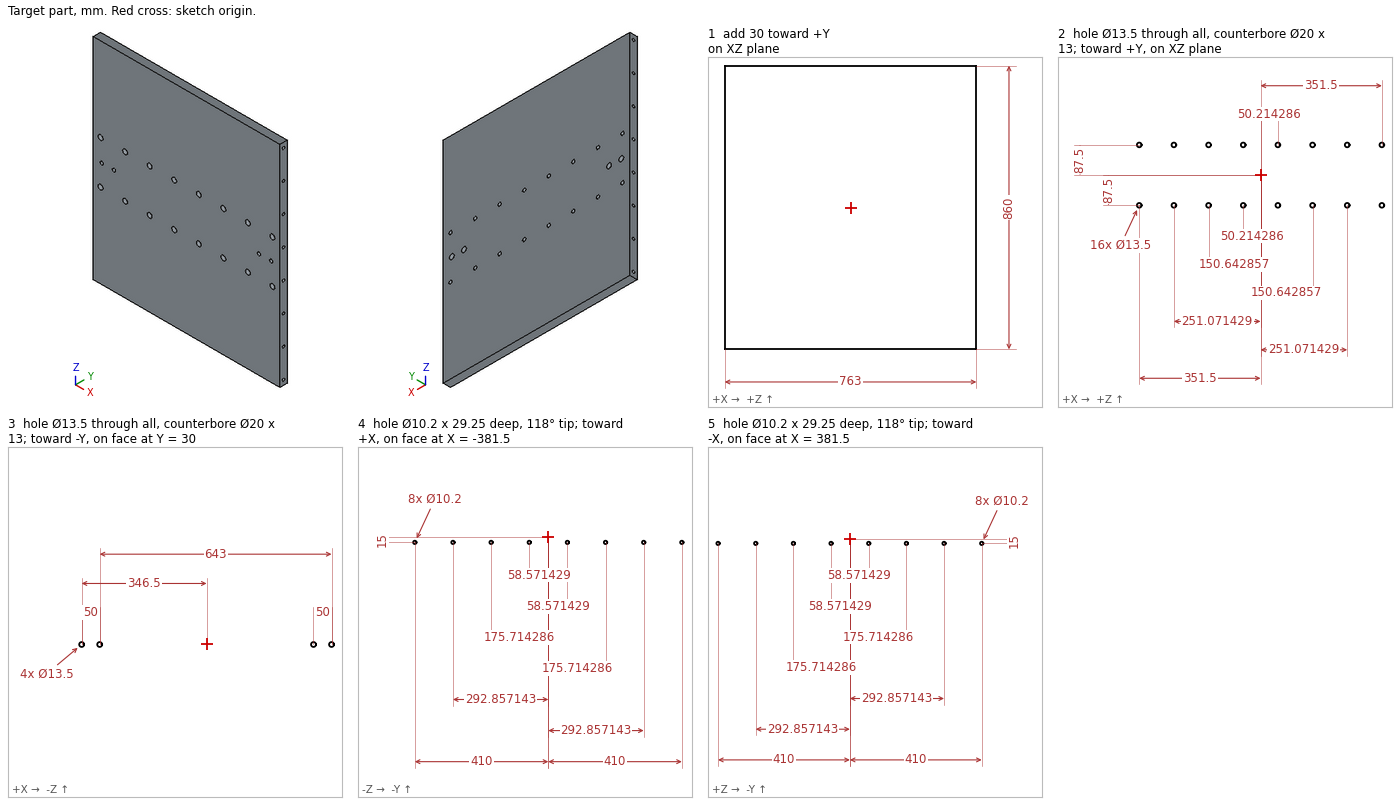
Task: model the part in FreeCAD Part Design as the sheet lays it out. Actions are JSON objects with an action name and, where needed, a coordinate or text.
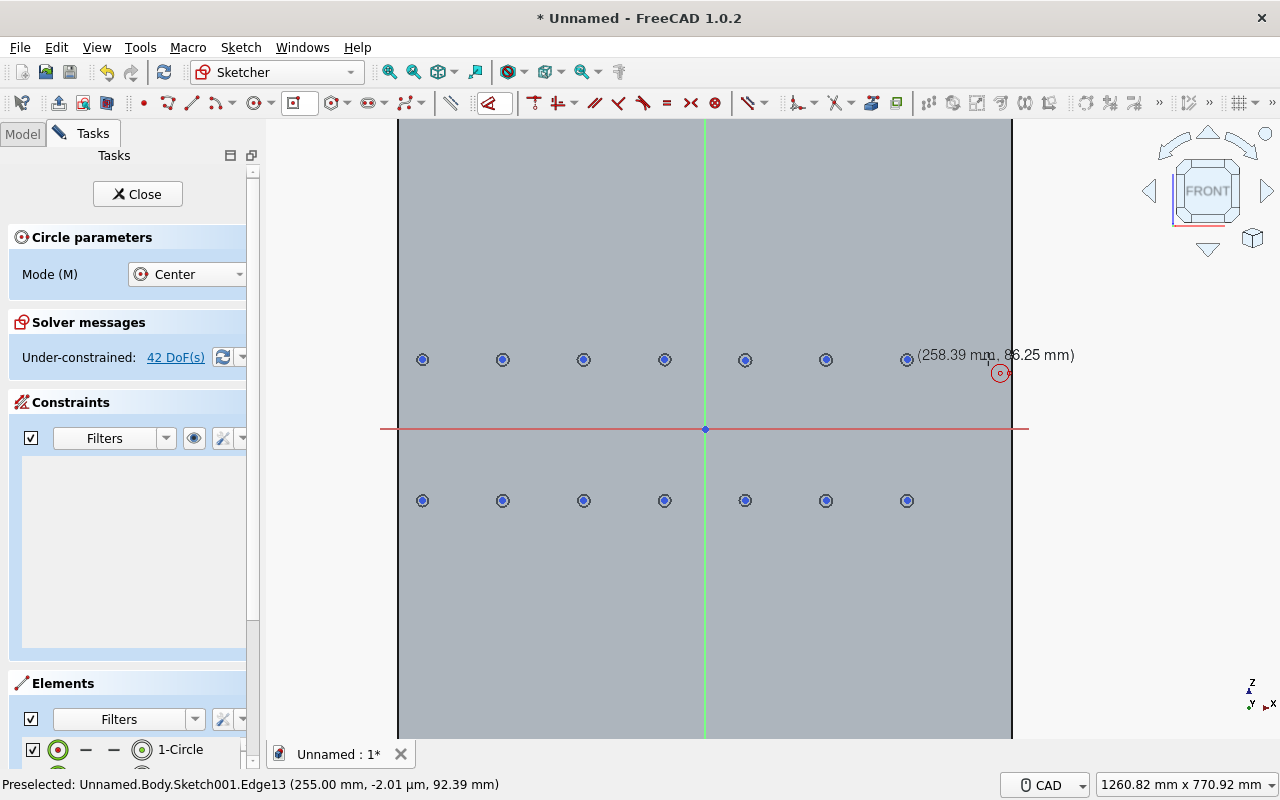
{"action": "left_click", "coordinate": [988, 359]}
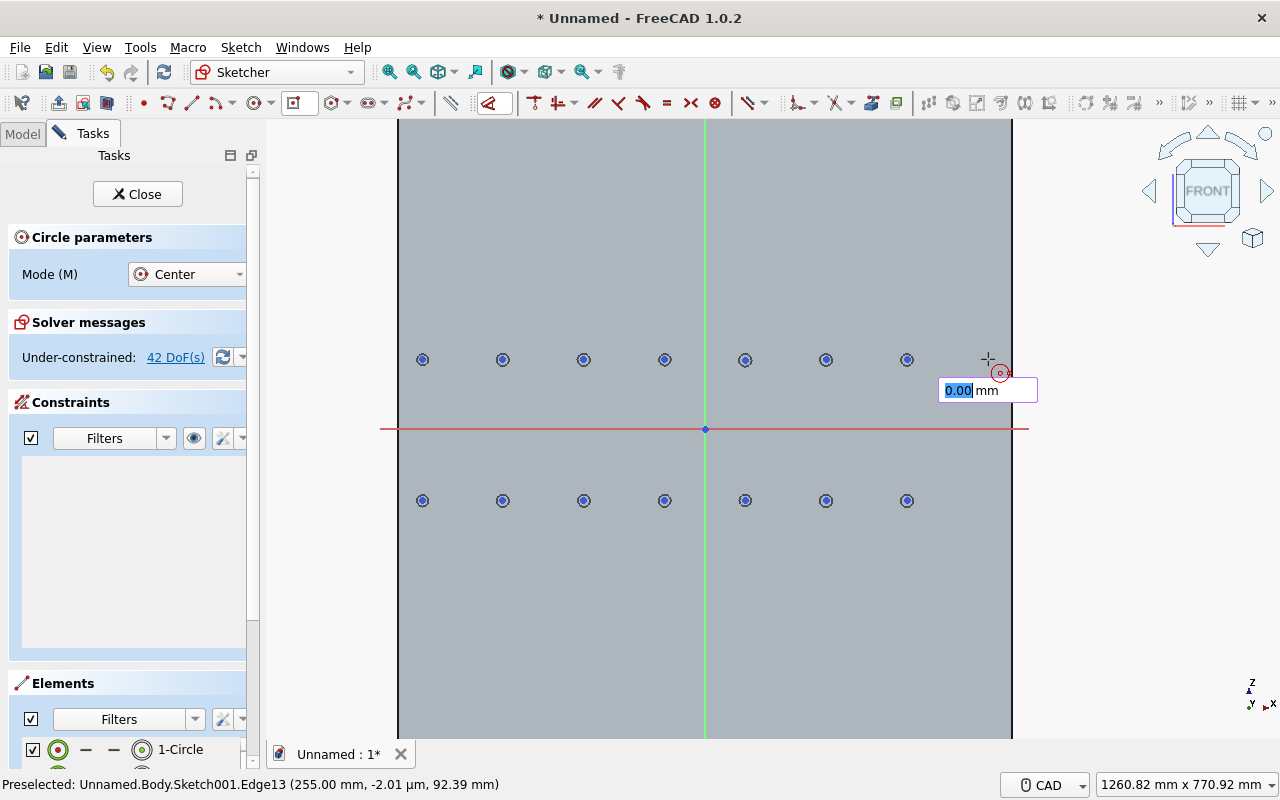
{"action": "scroll", "coordinate": [992, 355], "scroll_direction": "up", "scroll_amount": 6}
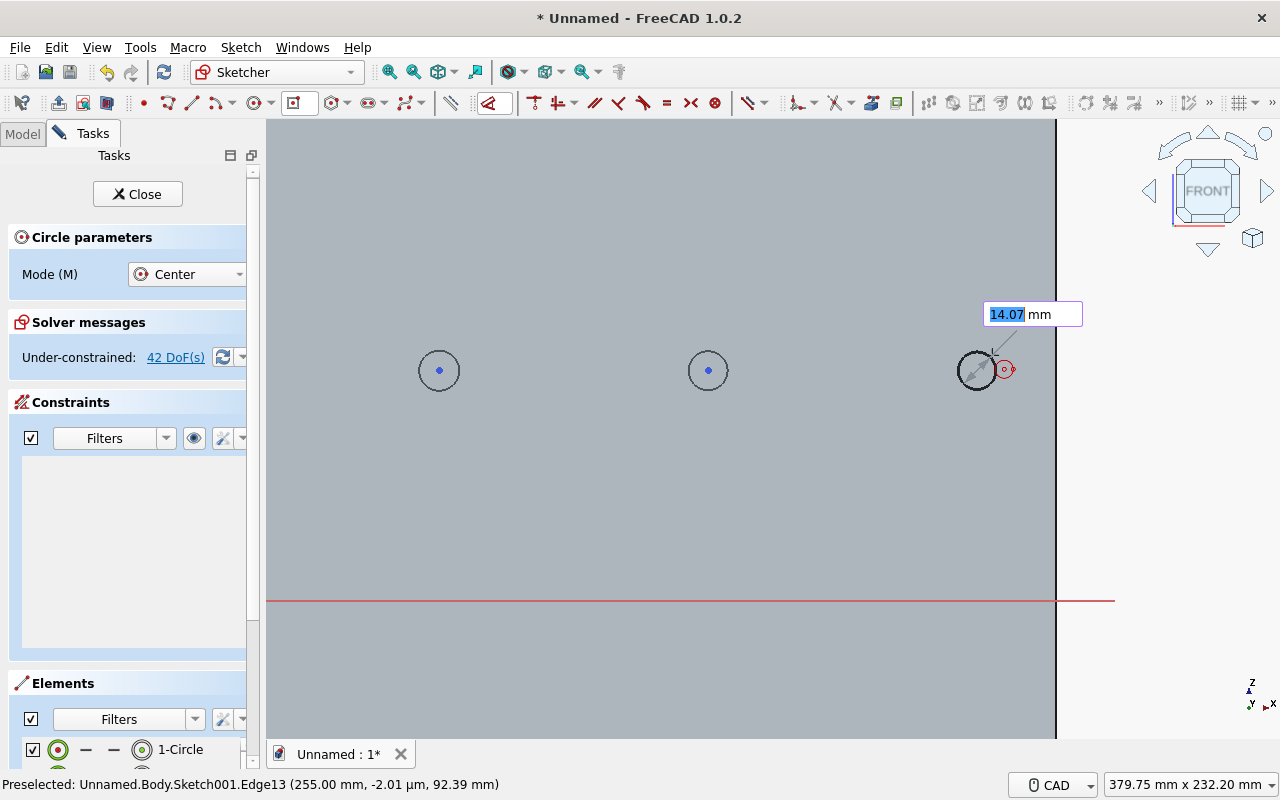
{"action": "left_click", "coordinate": [989, 355]}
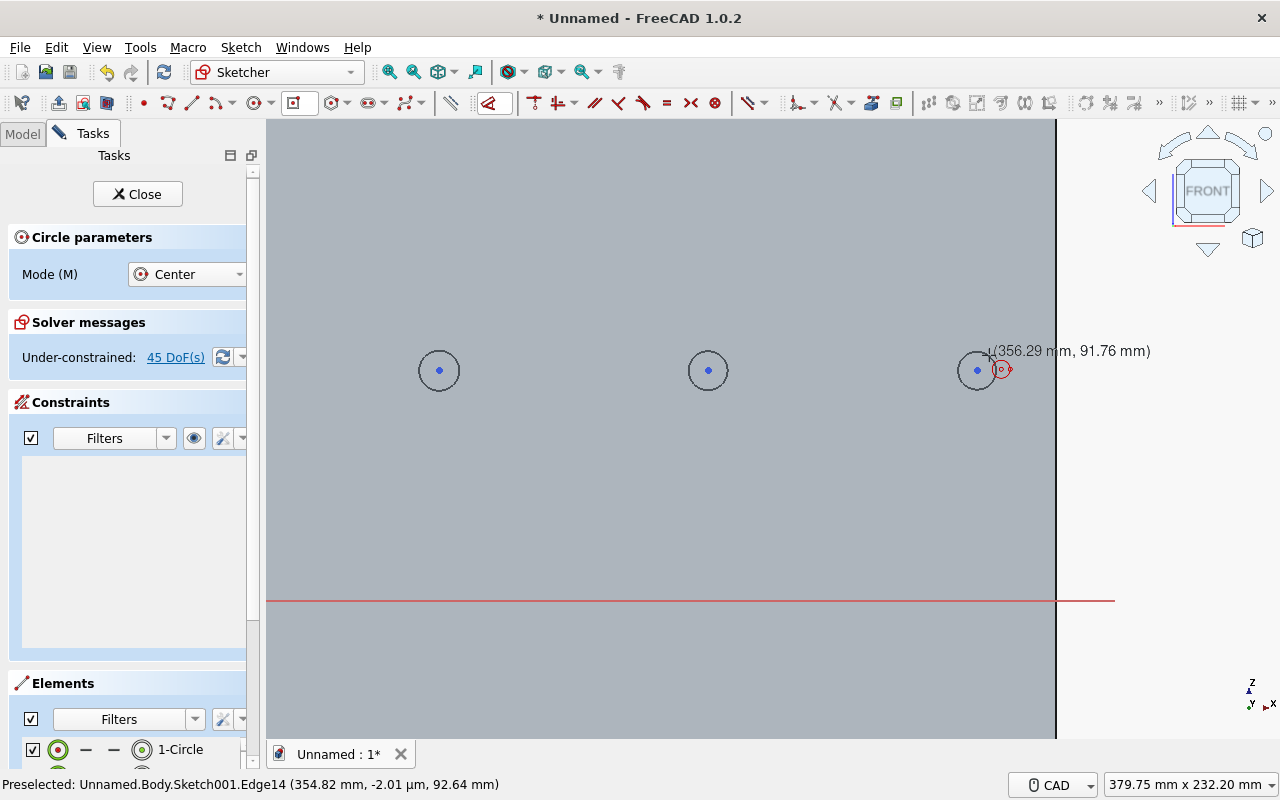
{"action": "scroll", "coordinate": [992, 355], "scroll_direction": "down", "scroll_amount": 6}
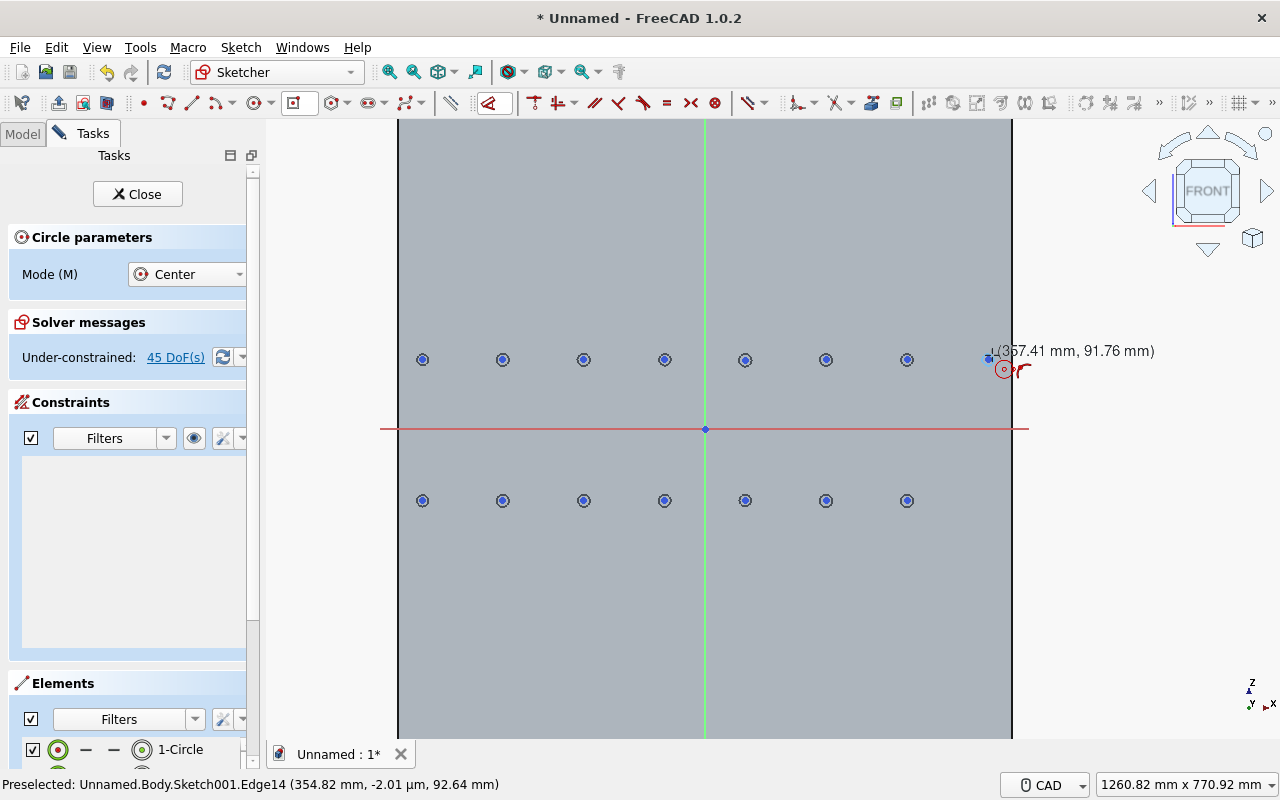
{"action": "scroll", "coordinate": [988, 500], "scroll_direction": "up", "scroll_amount": 8}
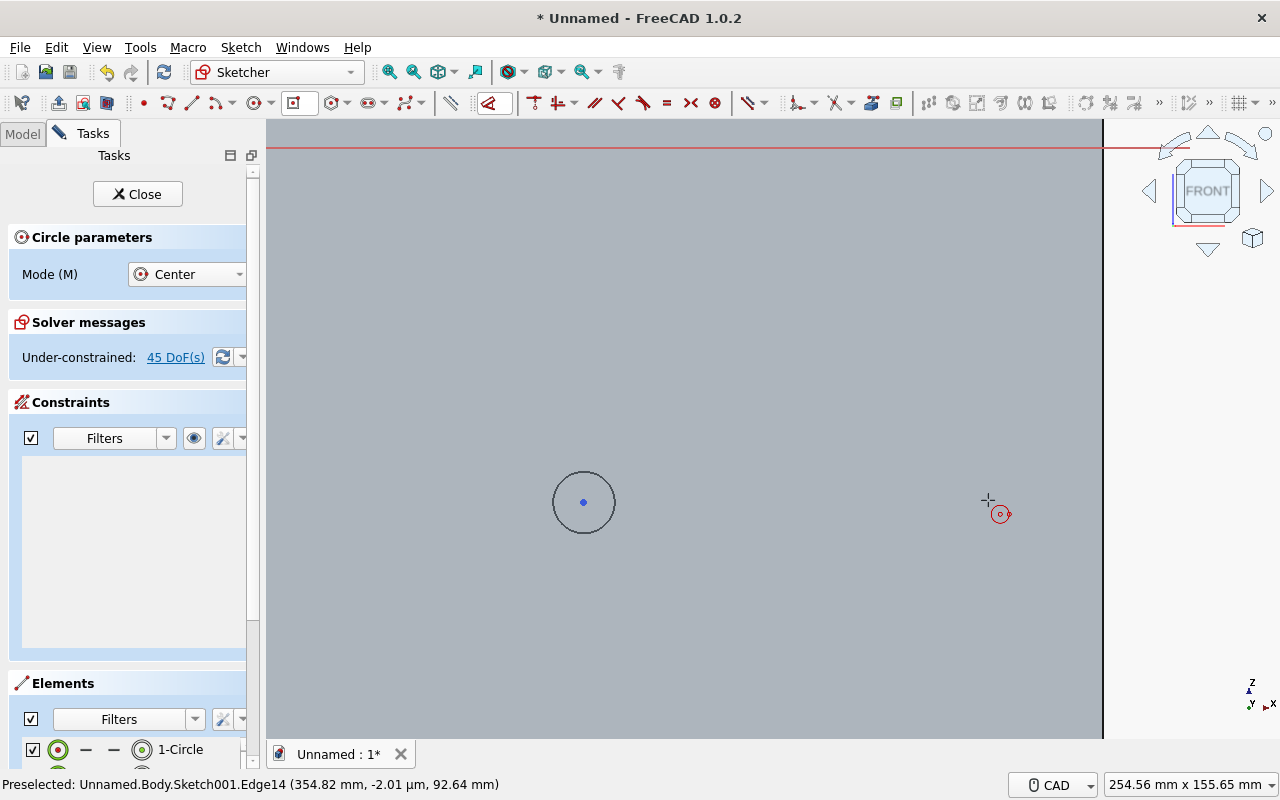
{"action": "scroll", "coordinate": [988, 500], "scroll_direction": "down", "scroll_amount": 8}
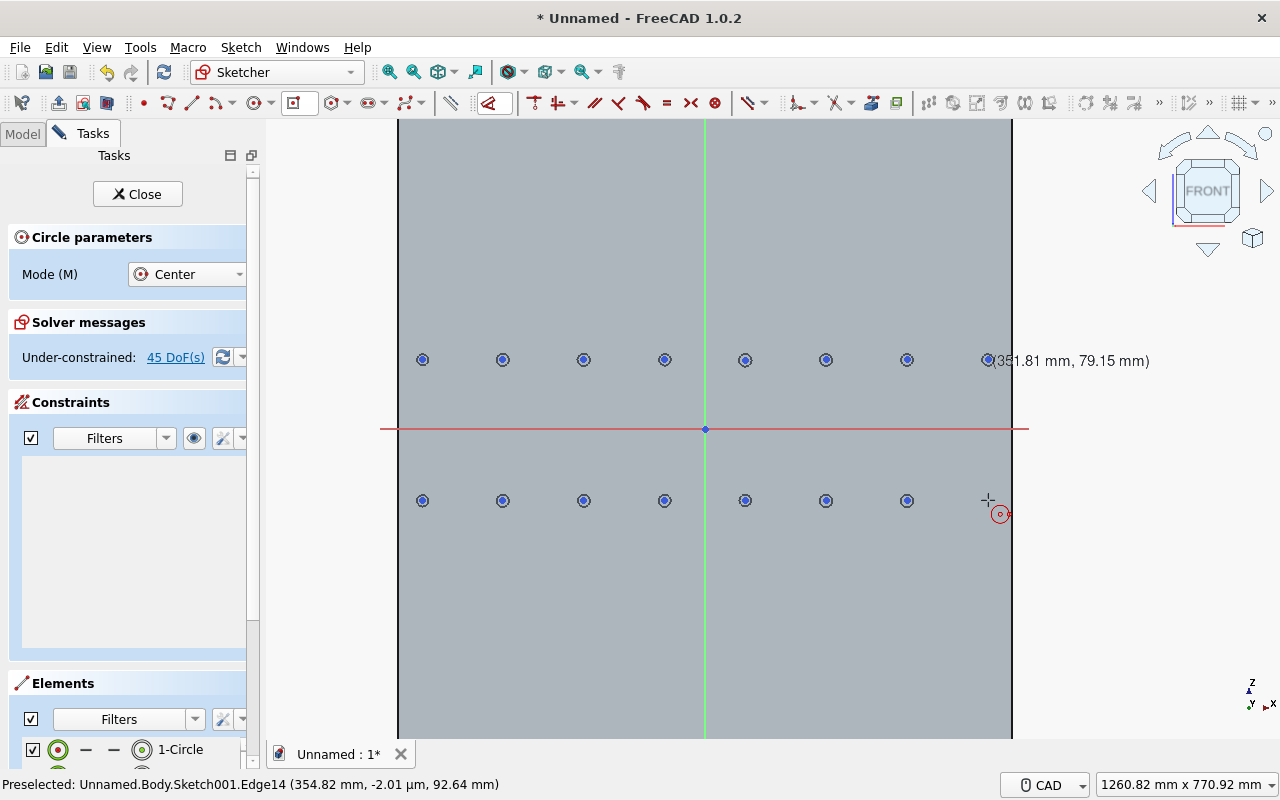
{"action": "left_click", "coordinate": [988, 500]}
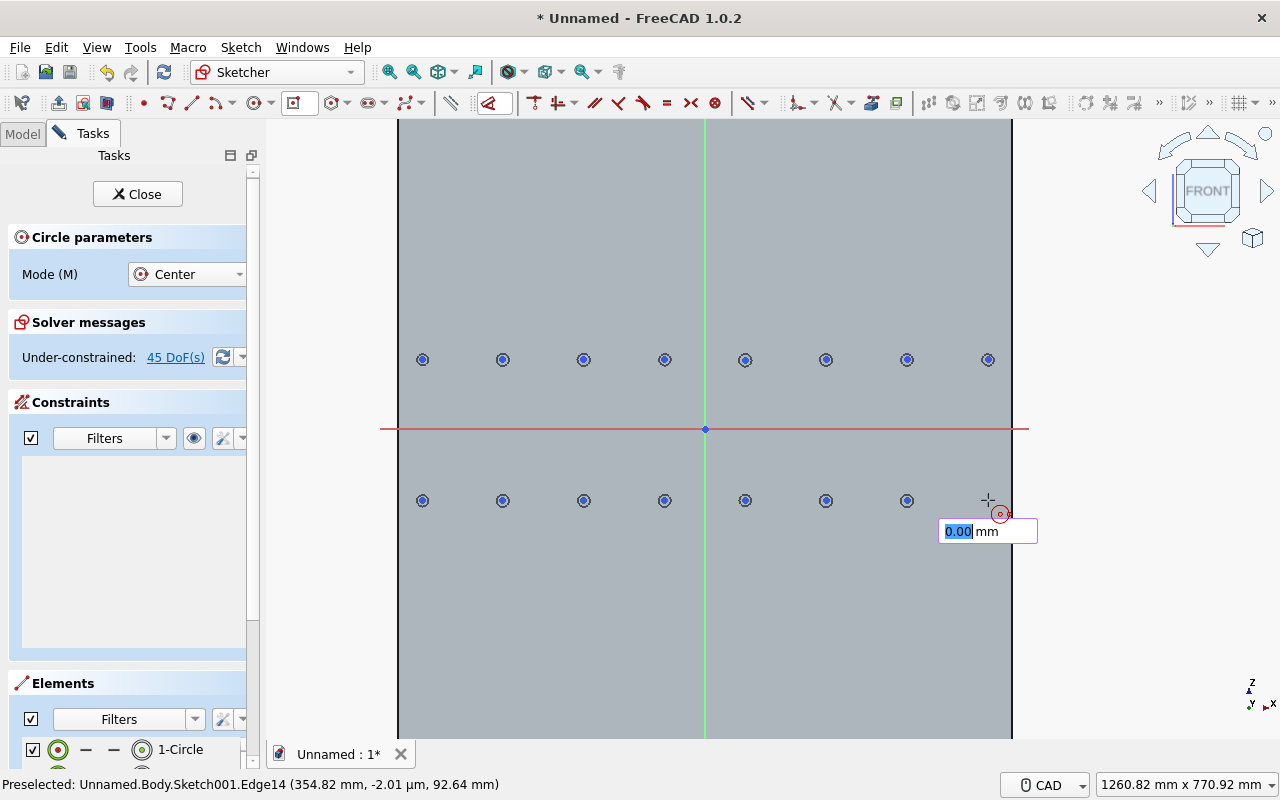
{"action": "scroll", "coordinate": [992, 496], "scroll_direction": "up", "scroll_amount": 6}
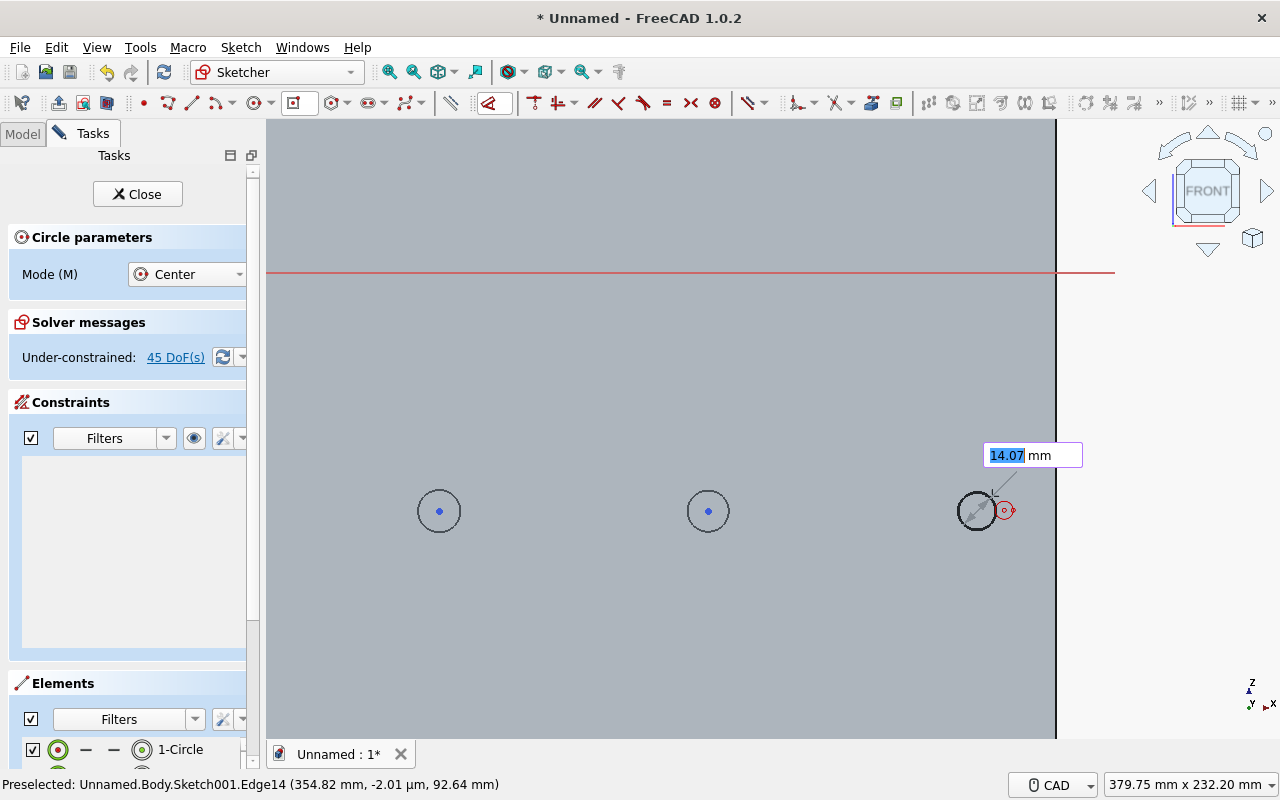
{"action": "left_click", "coordinate": [989, 494]}
{"action": "key", "text": "Escape"}